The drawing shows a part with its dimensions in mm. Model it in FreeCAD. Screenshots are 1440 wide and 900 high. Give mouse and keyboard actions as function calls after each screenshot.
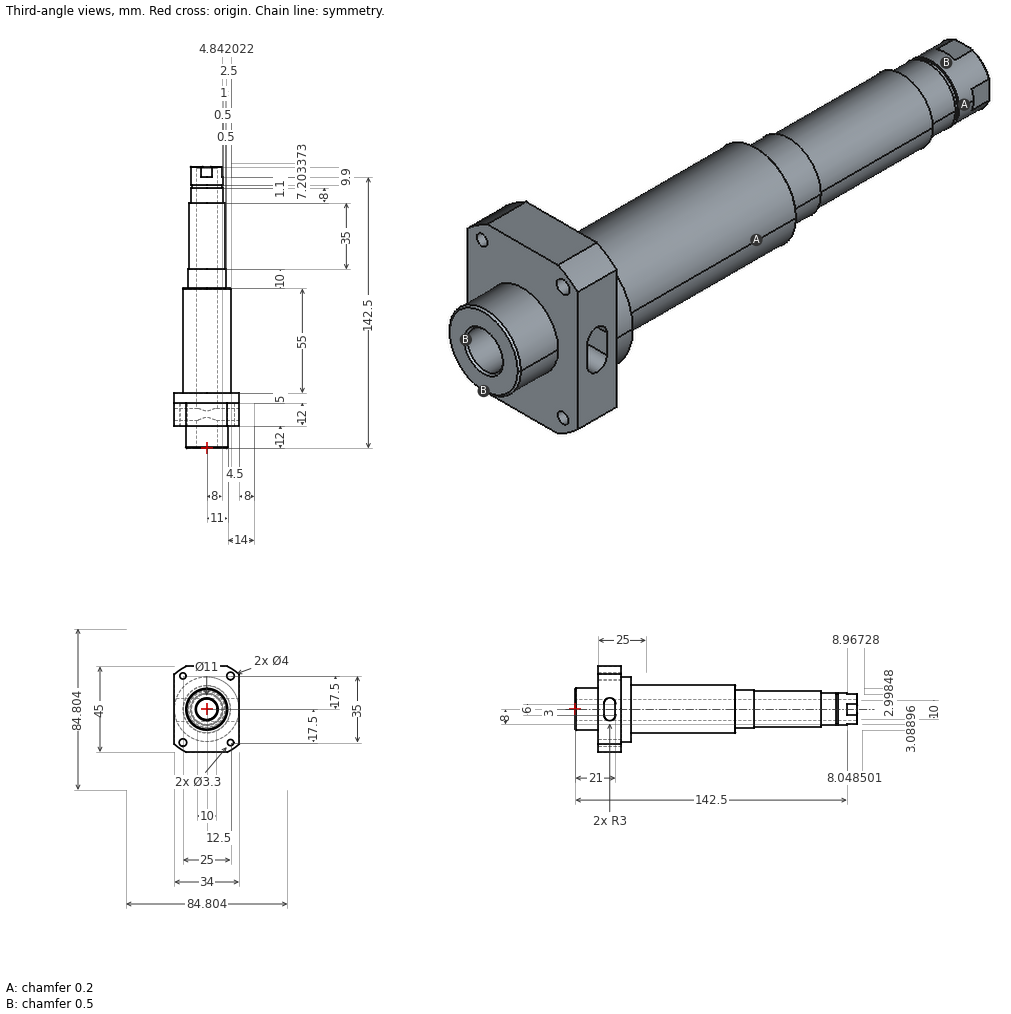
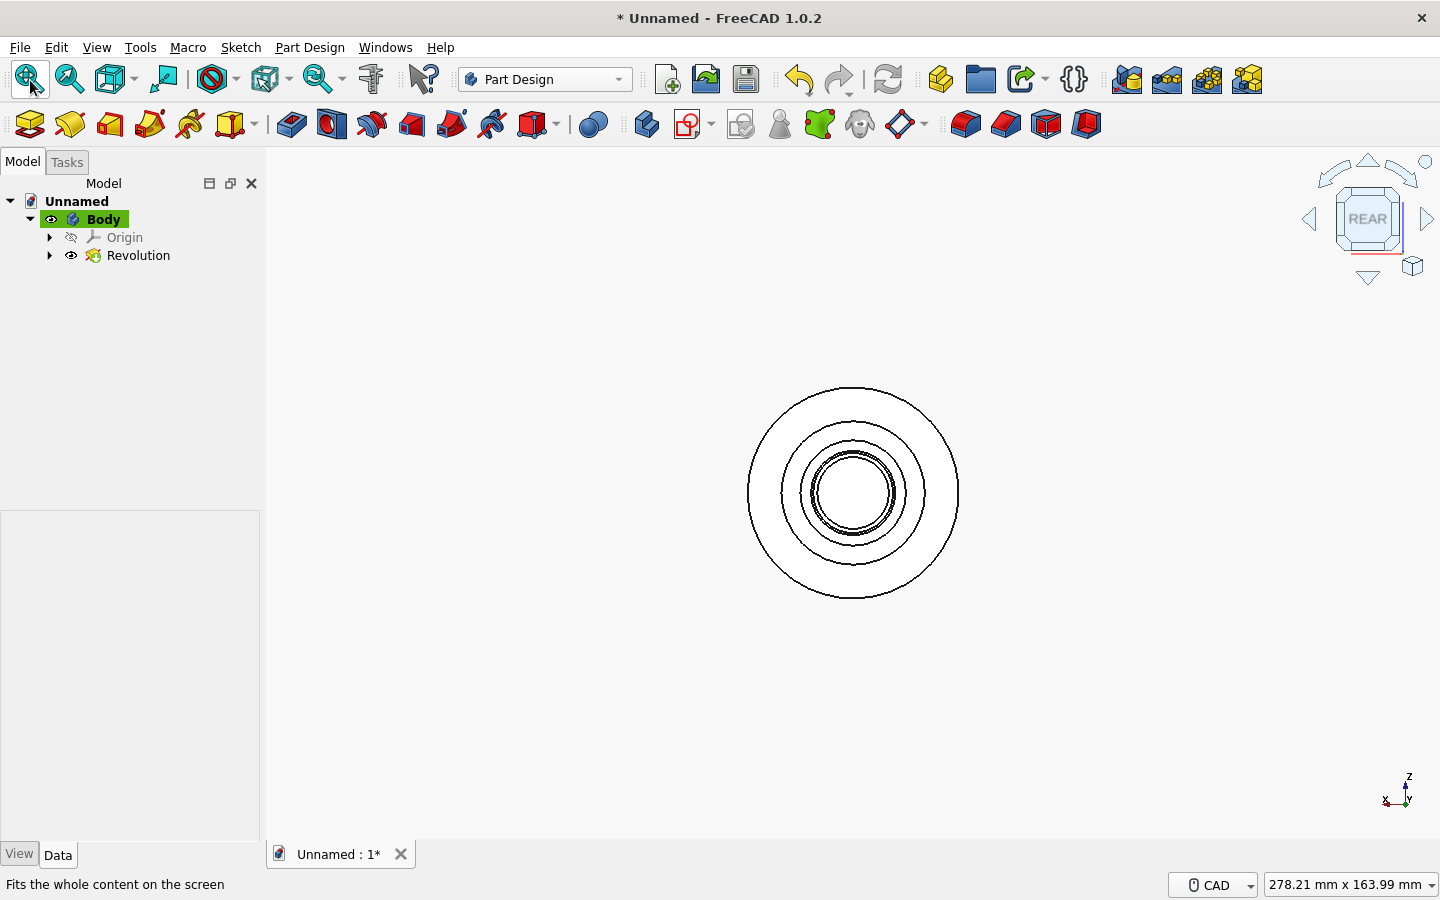
click(853, 582)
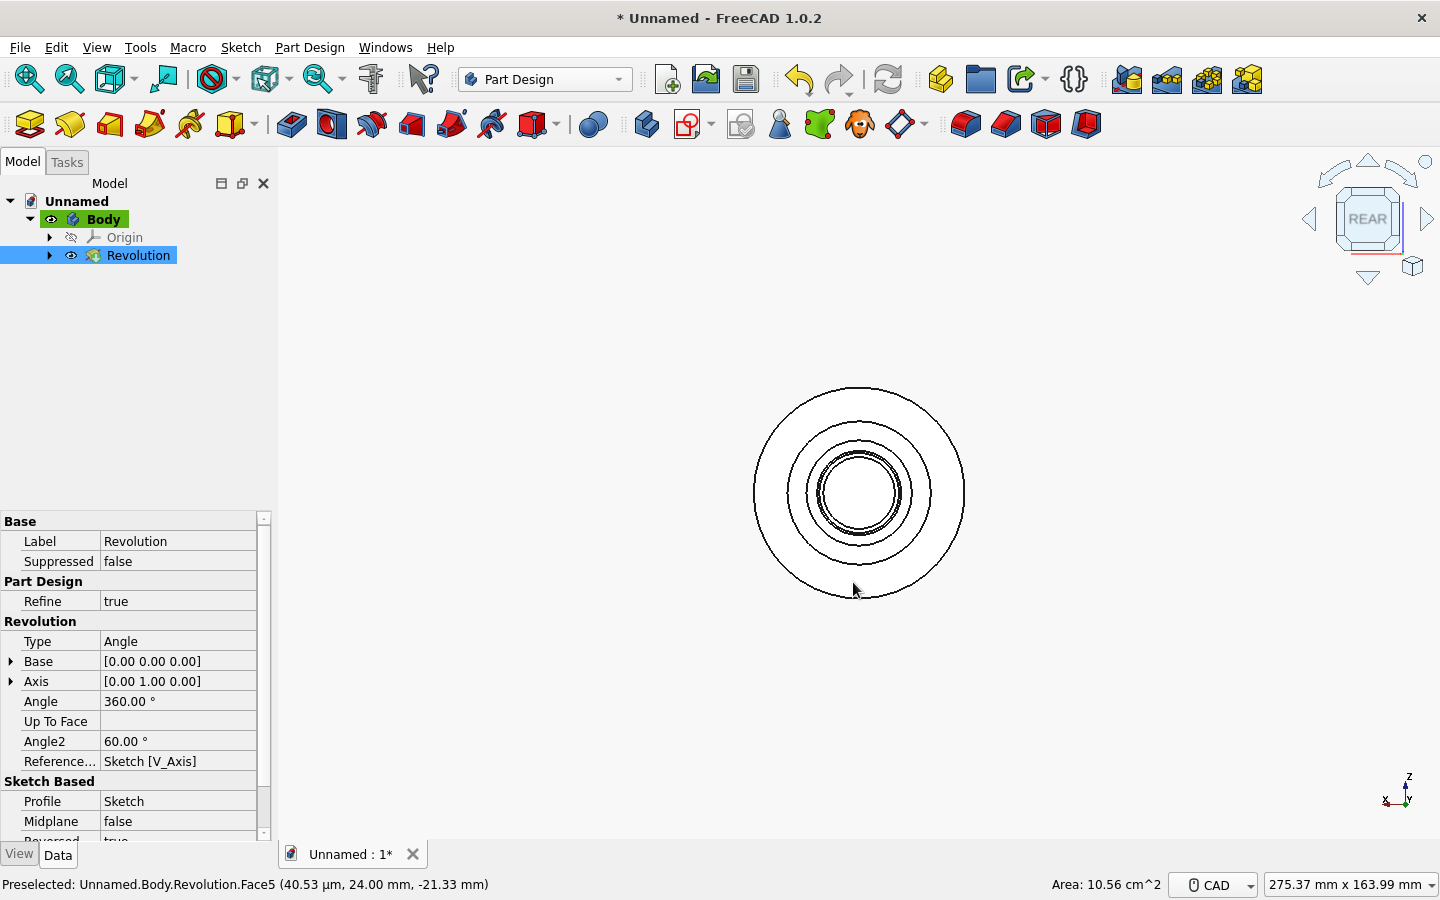
click(688, 124)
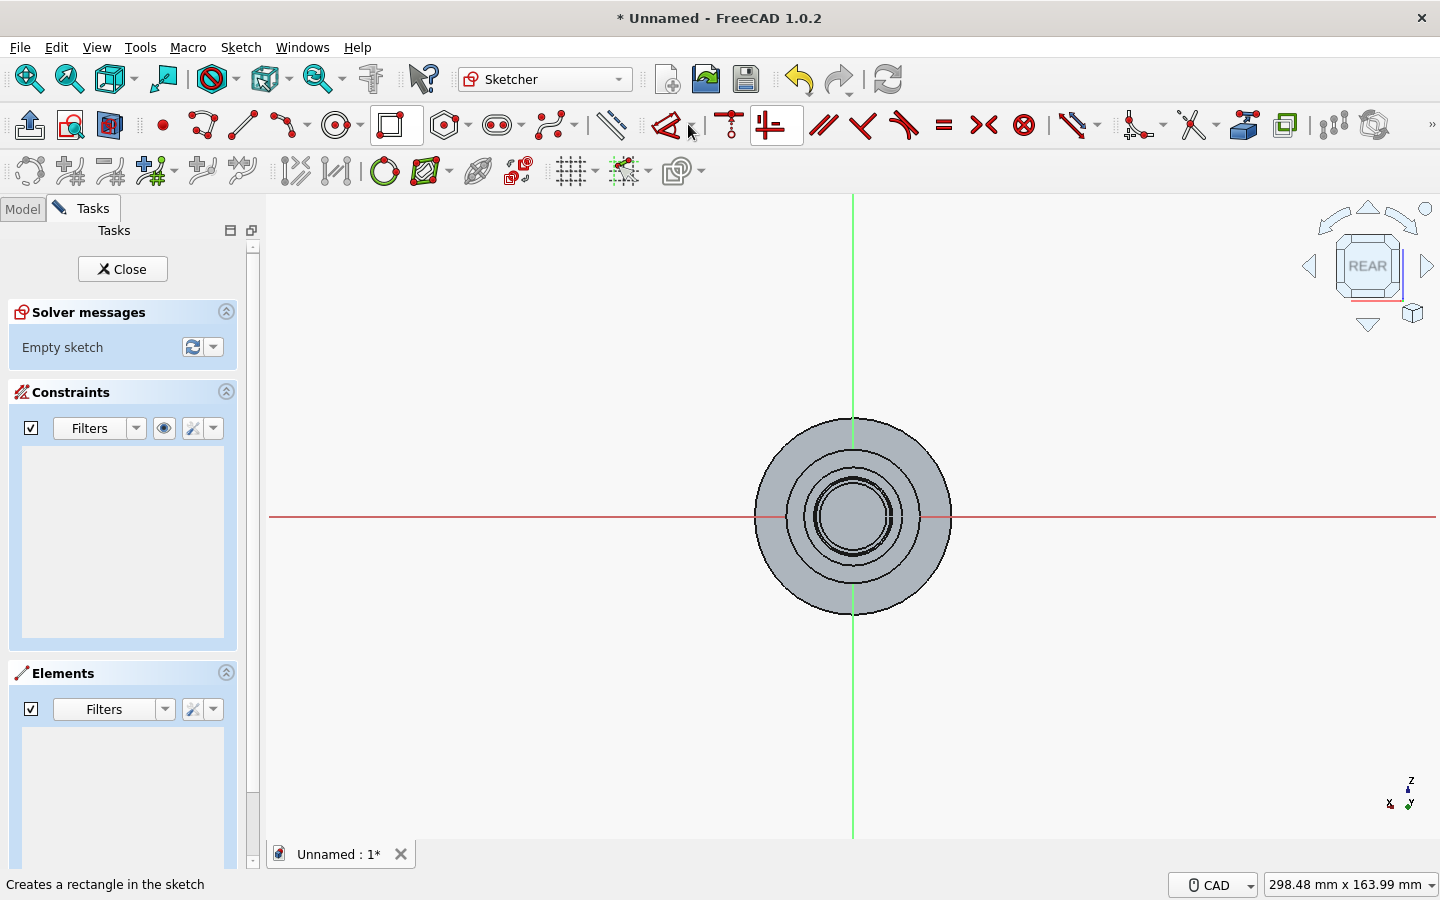
click(418, 126)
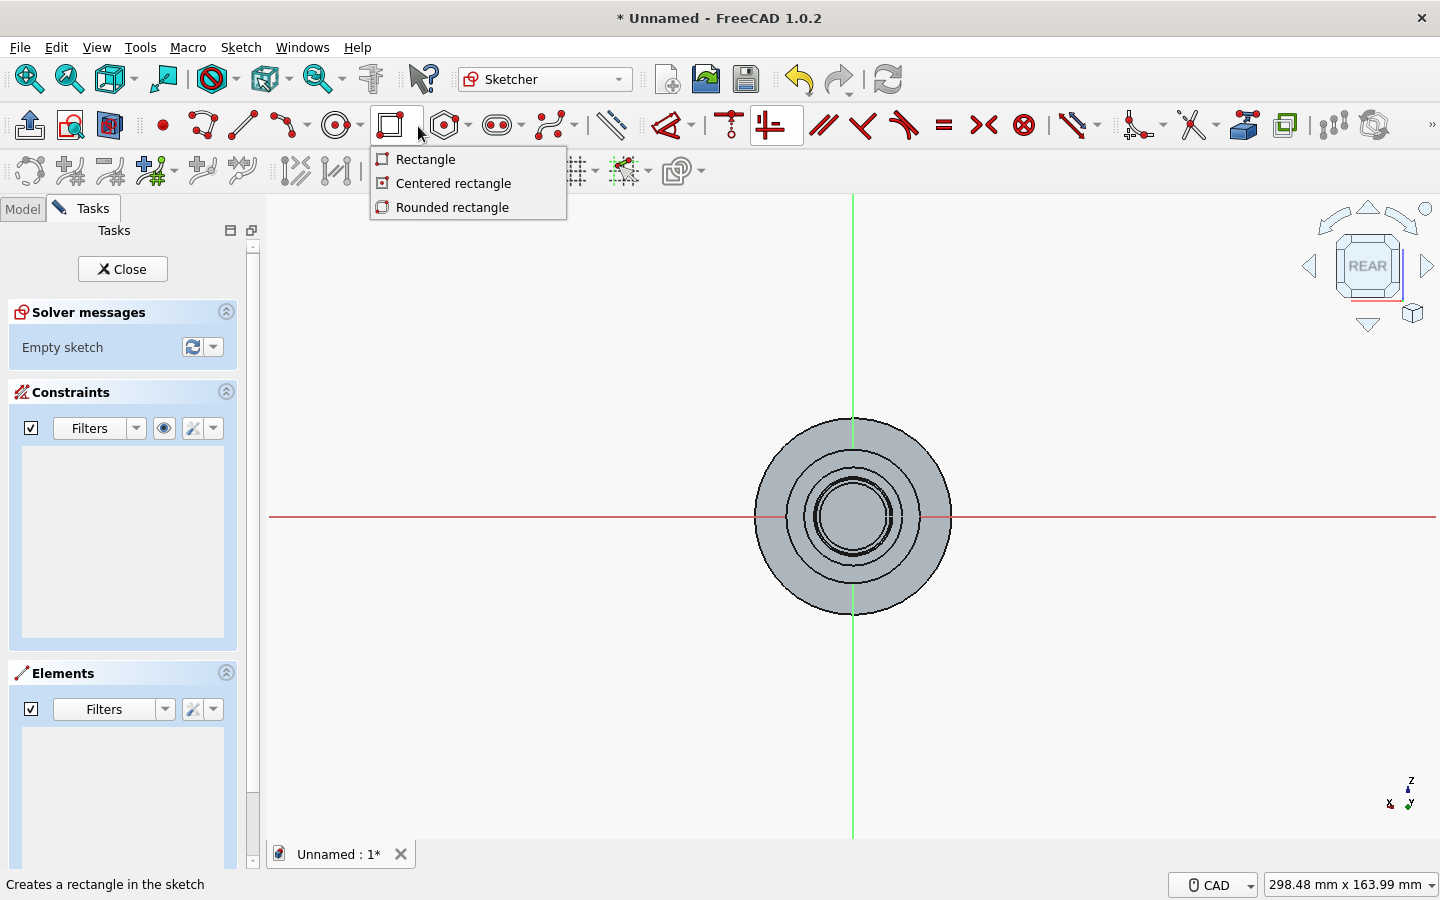
click(468, 183)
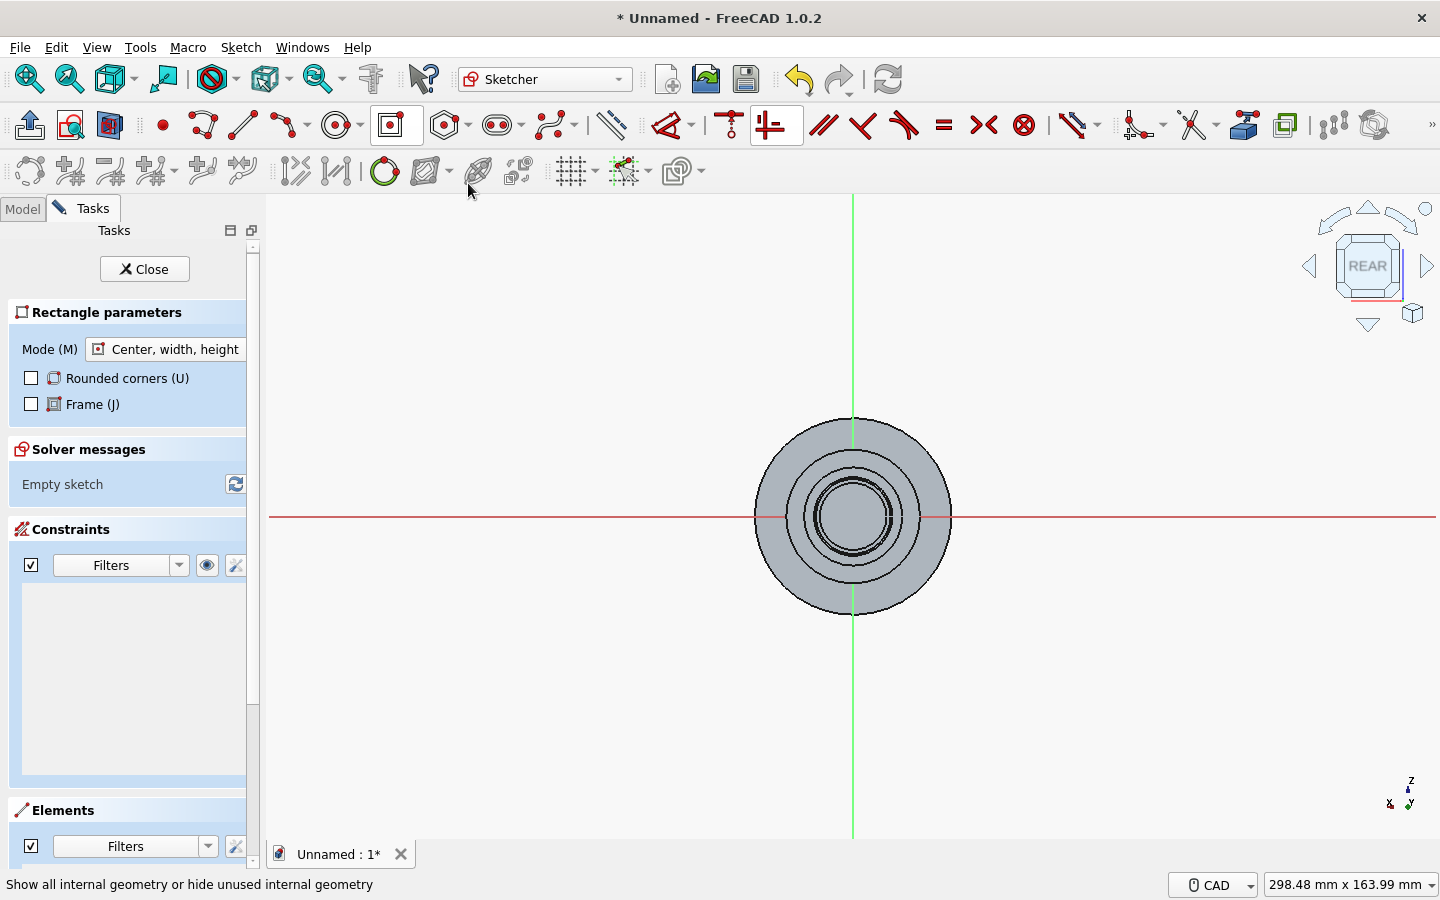
click(853, 516)
move(1020, 350)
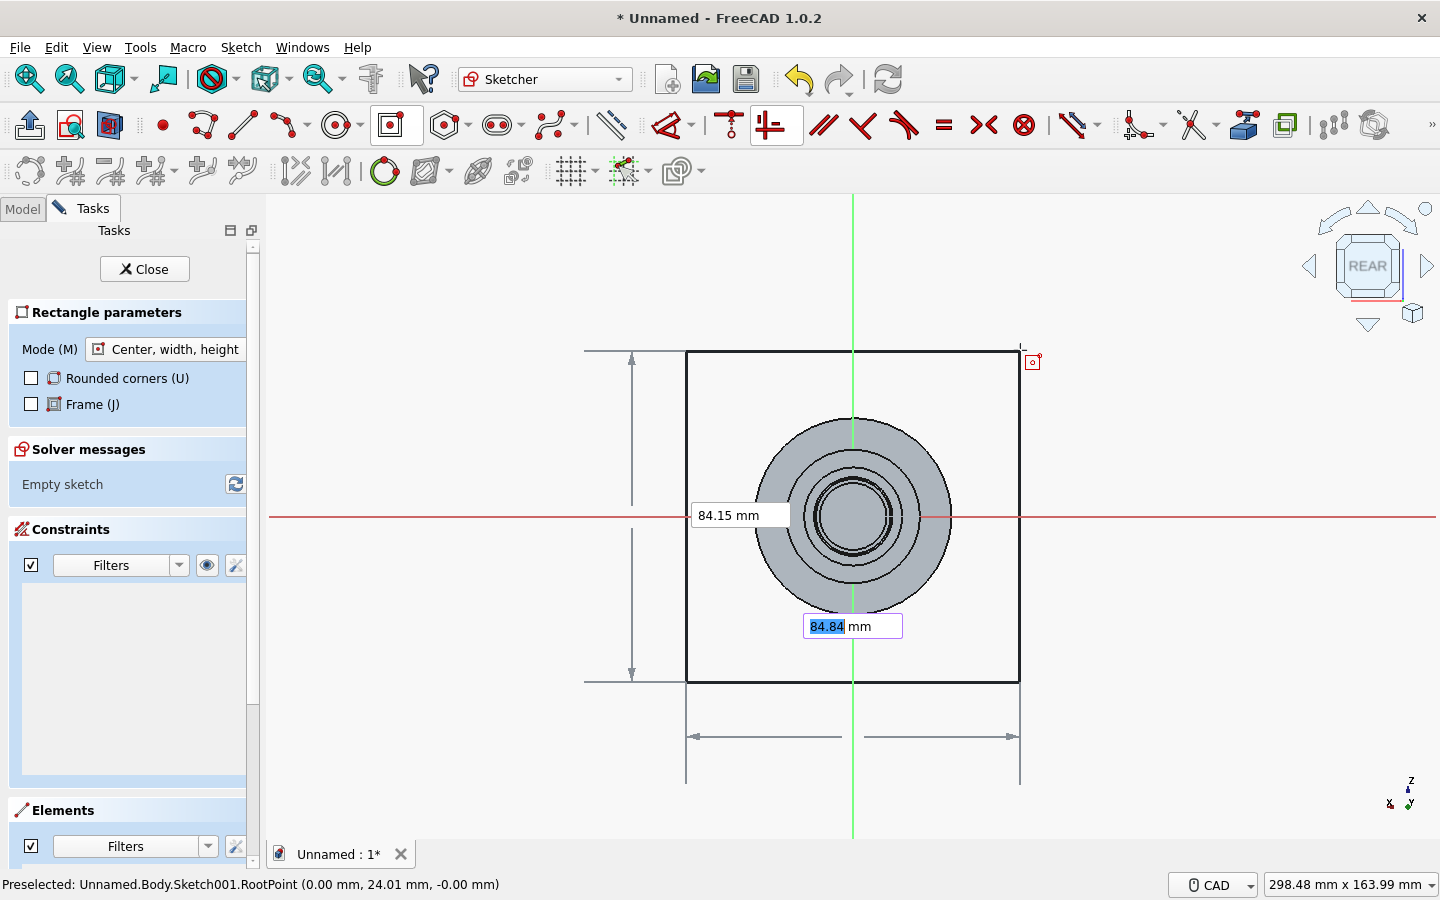
text(84.804)
key(Tab)
text(84.804)
key(Return)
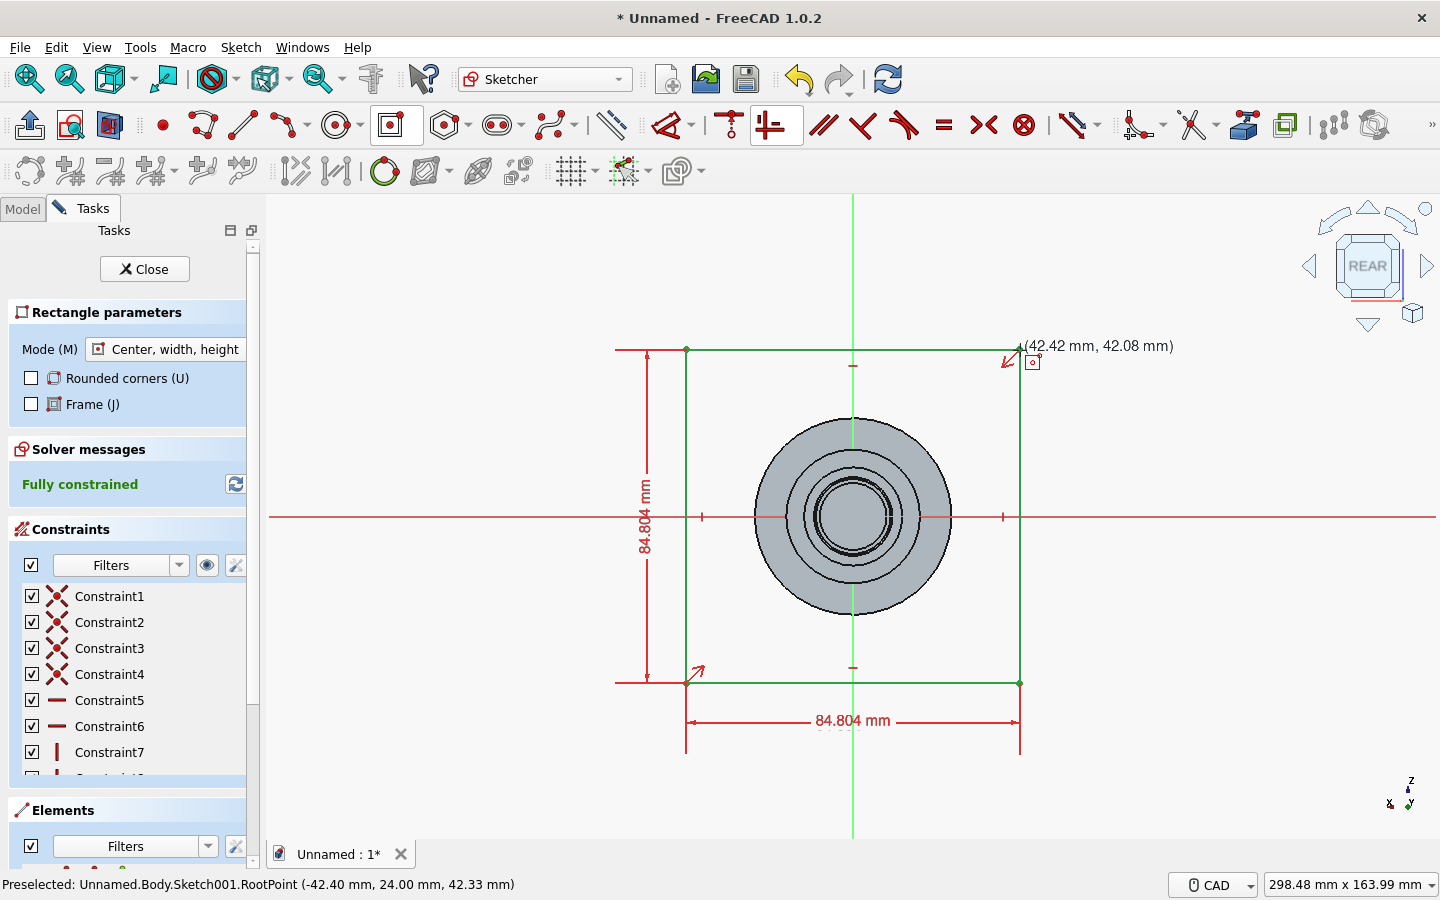
click(853, 516)
move(920, 428)